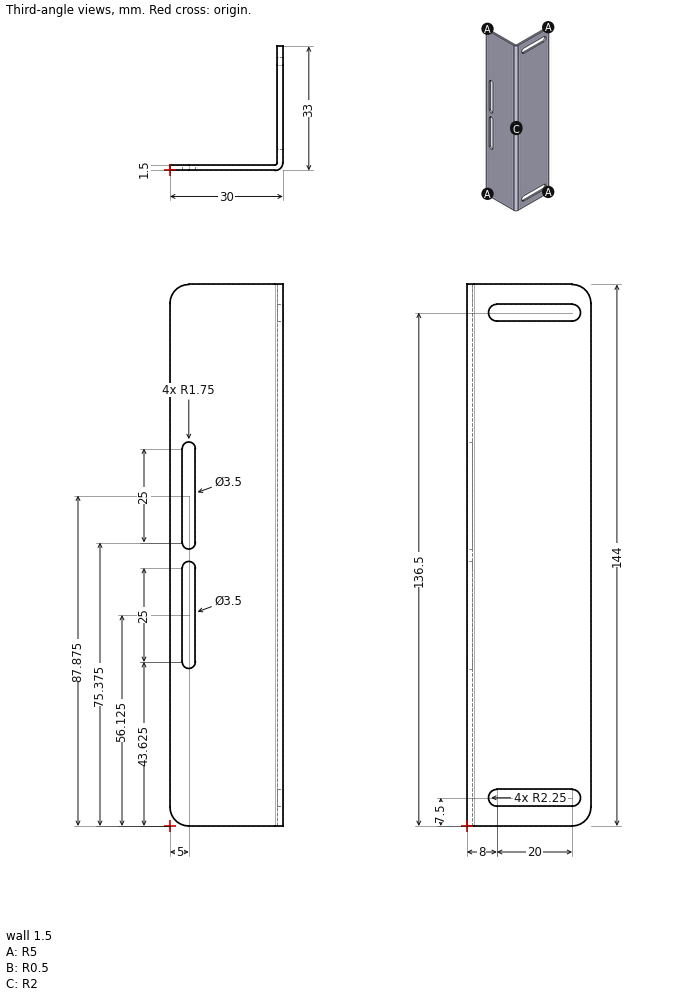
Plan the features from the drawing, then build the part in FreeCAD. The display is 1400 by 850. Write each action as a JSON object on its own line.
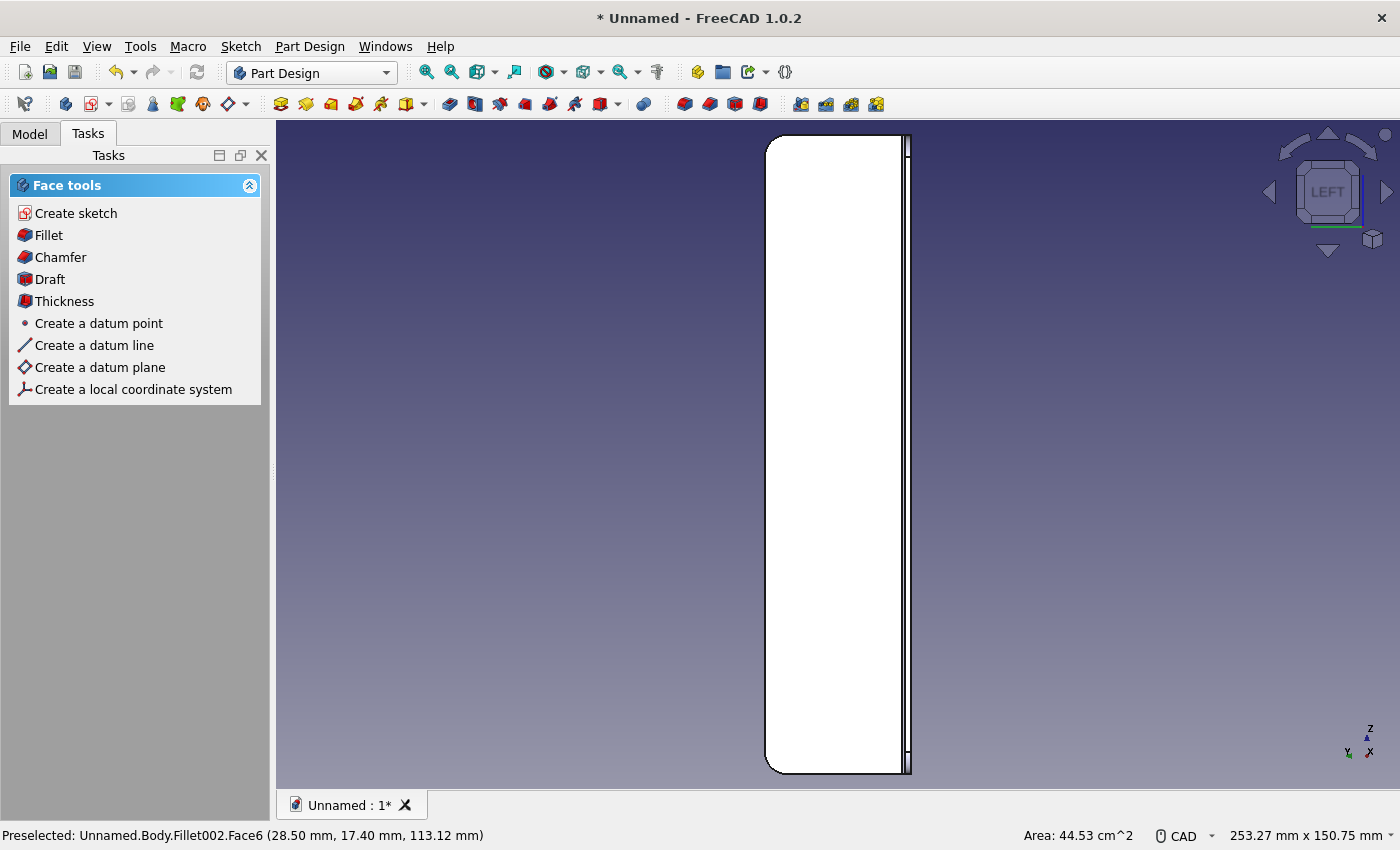
{"action": "left_click", "coordinate": [90, 104]}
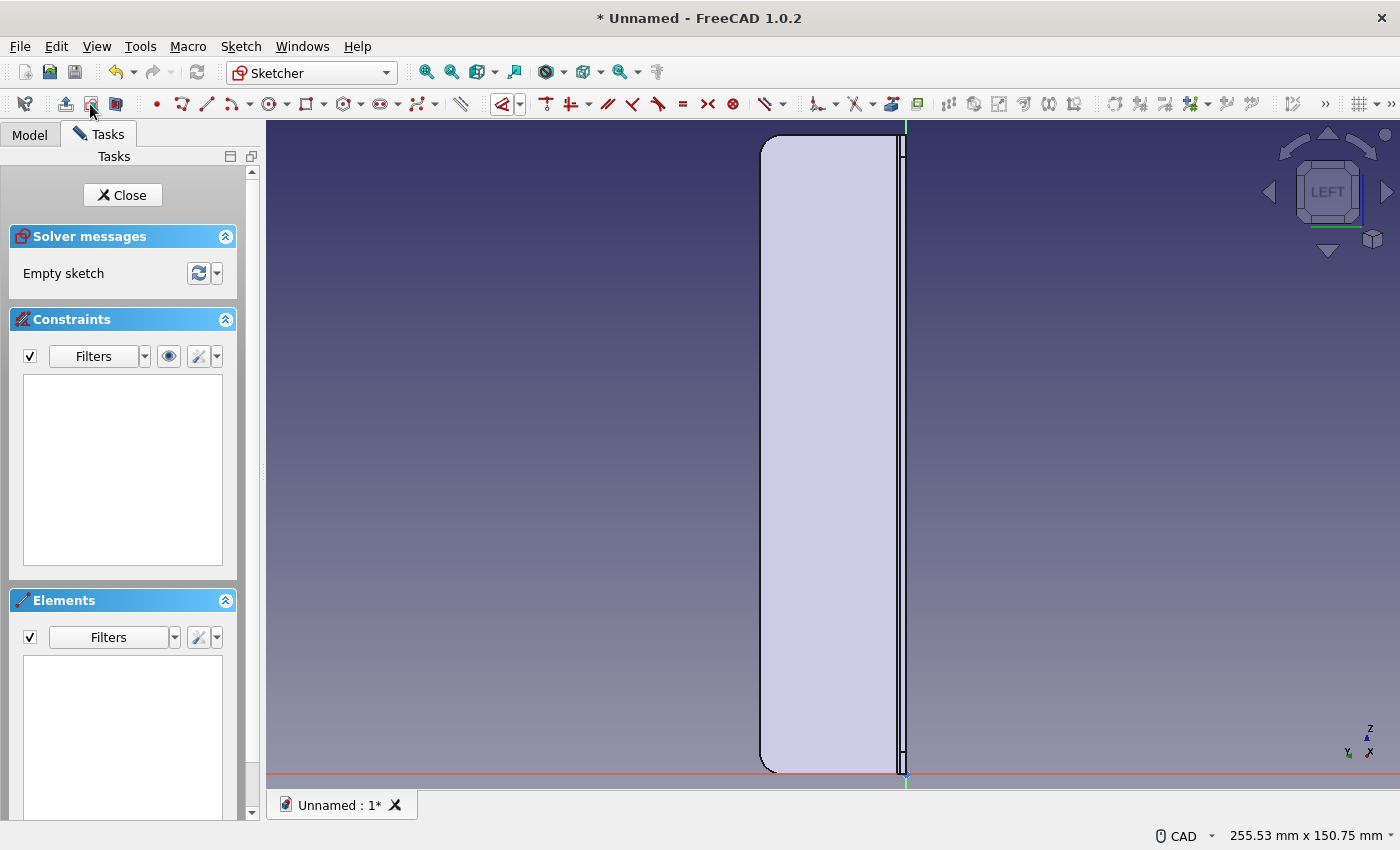
{"action": "left_click", "coordinate": [116, 104]}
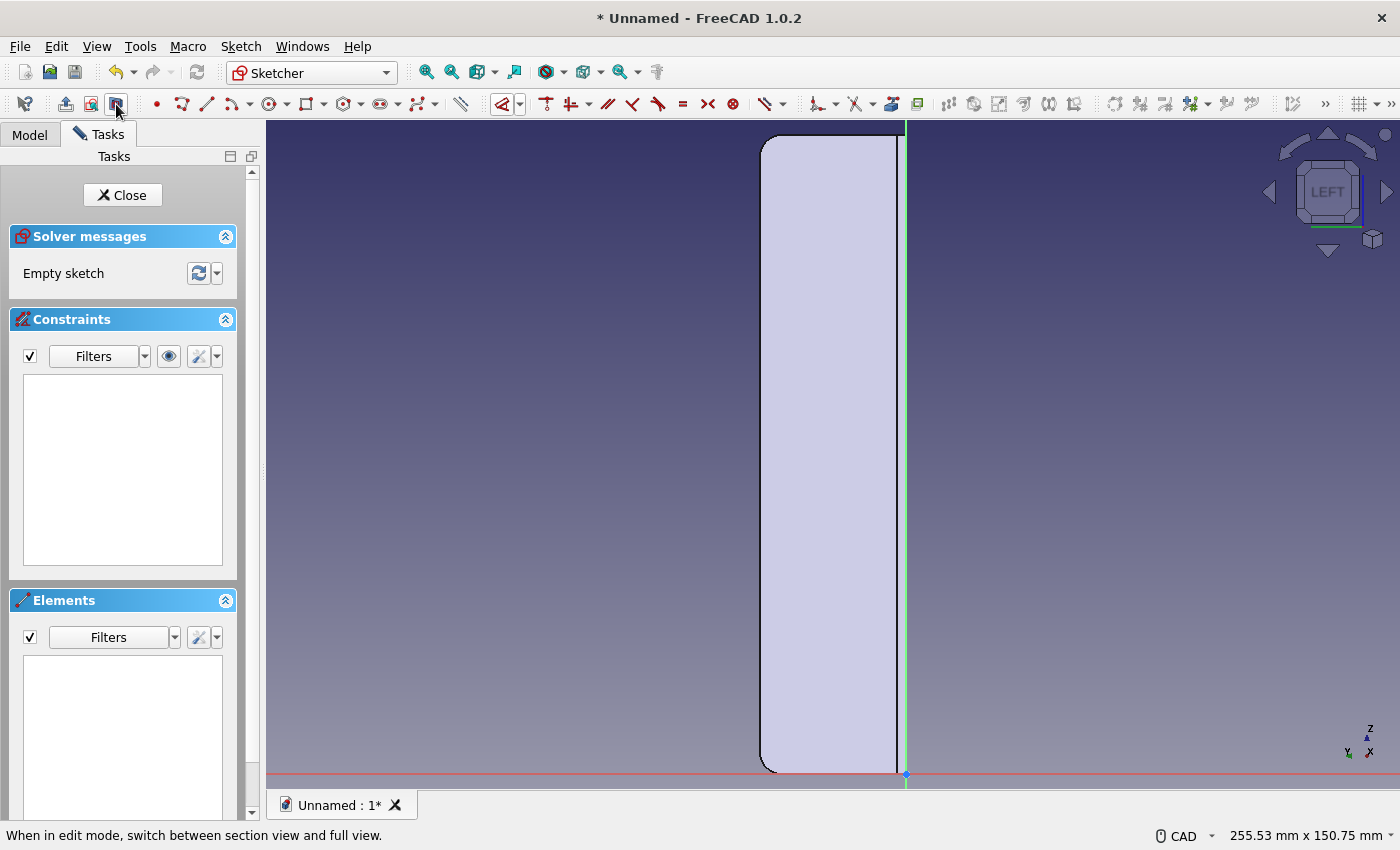
{"action": "scroll", "coordinate": [613, 431], "scroll_direction": "down", "scroll_amount": 2}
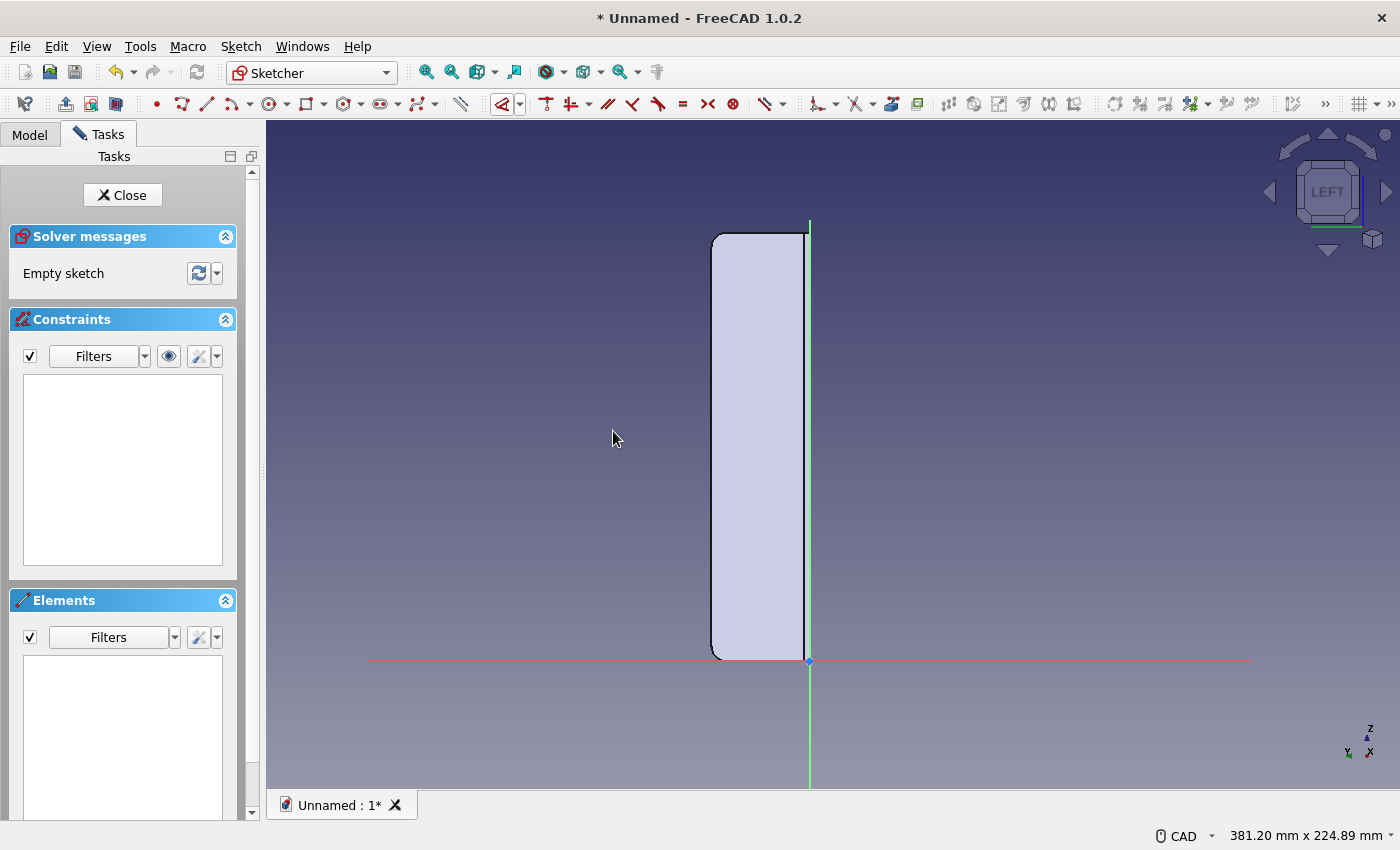
{"action": "left_click", "coordinate": [380, 104]}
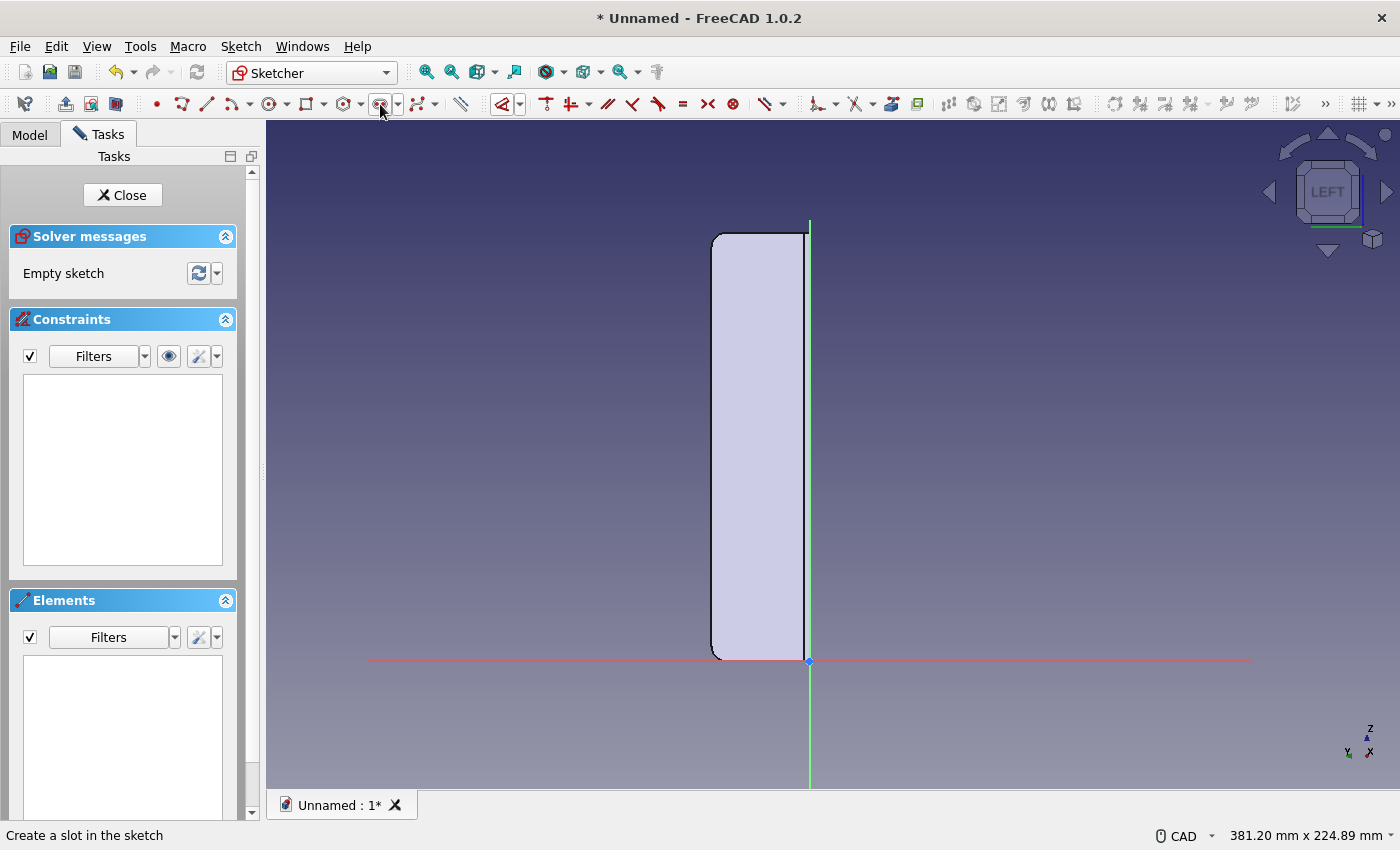
{"action": "scroll", "coordinate": [726, 639], "scroll_direction": "up", "scroll_amount": 7}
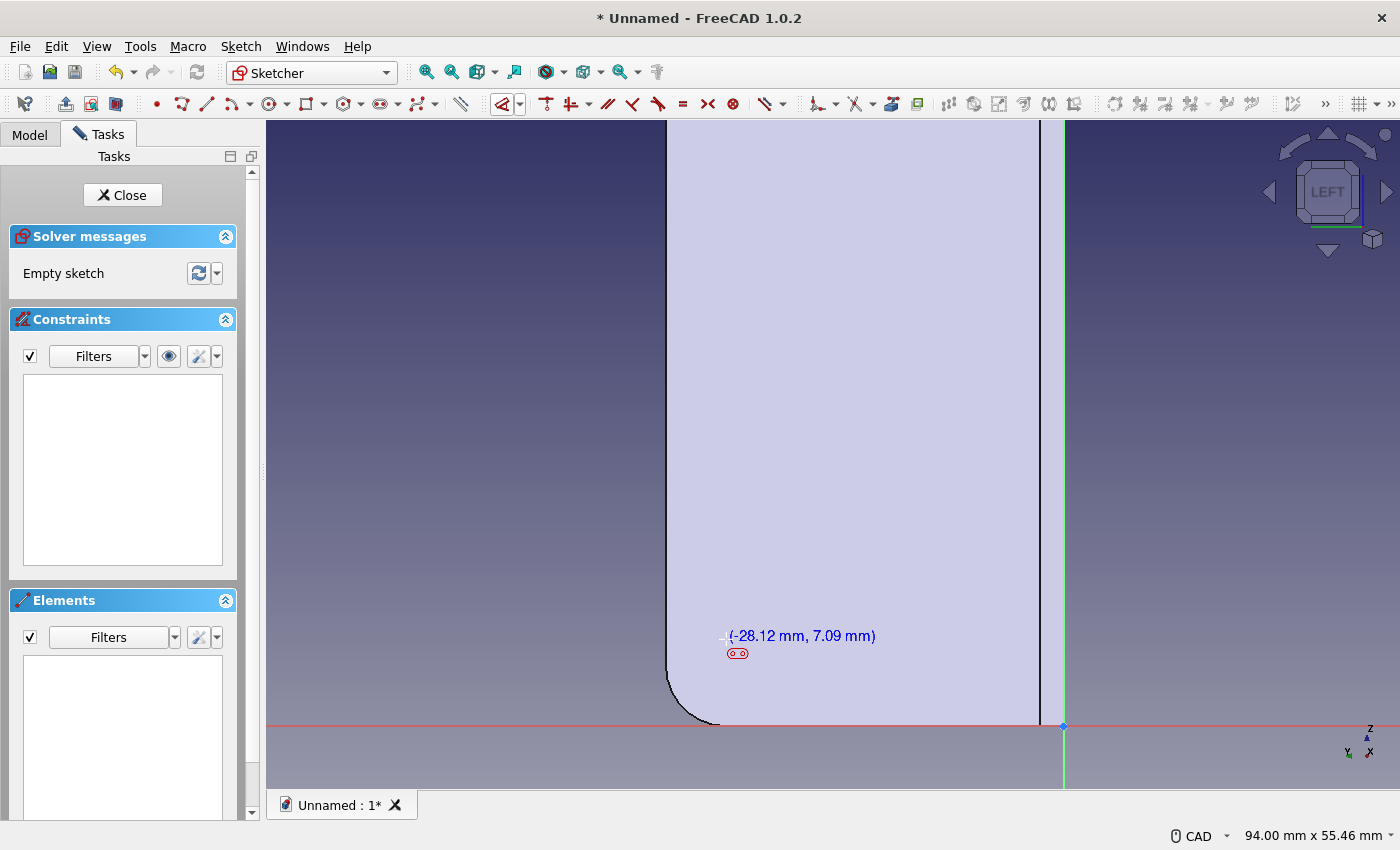
{"action": "scroll", "coordinate": [726, 639], "scroll_direction": "down", "scroll_amount": 7}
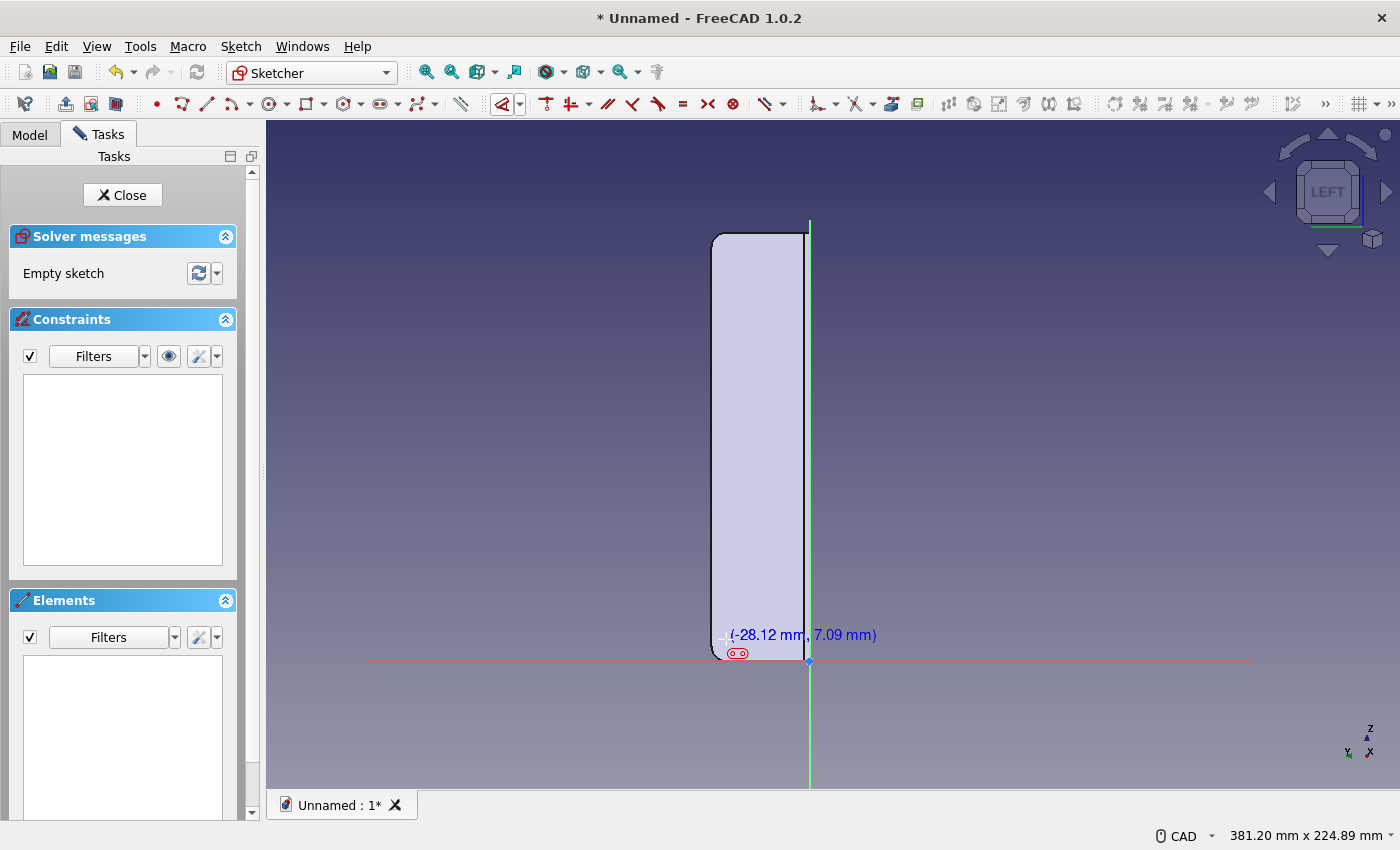
{"action": "left_click", "coordinate": [726, 639]}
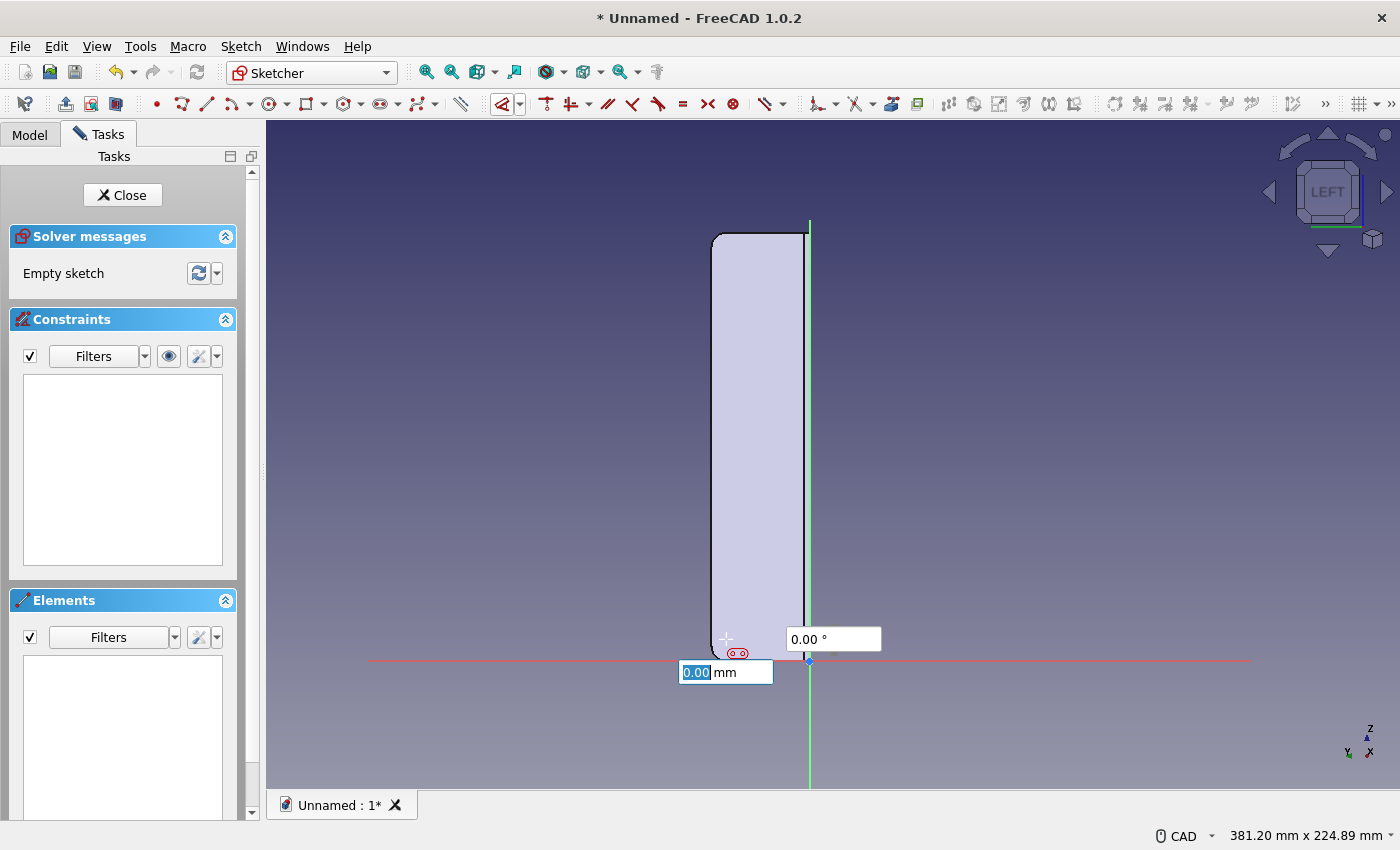
{"action": "left_click", "coordinate": [786, 639]}